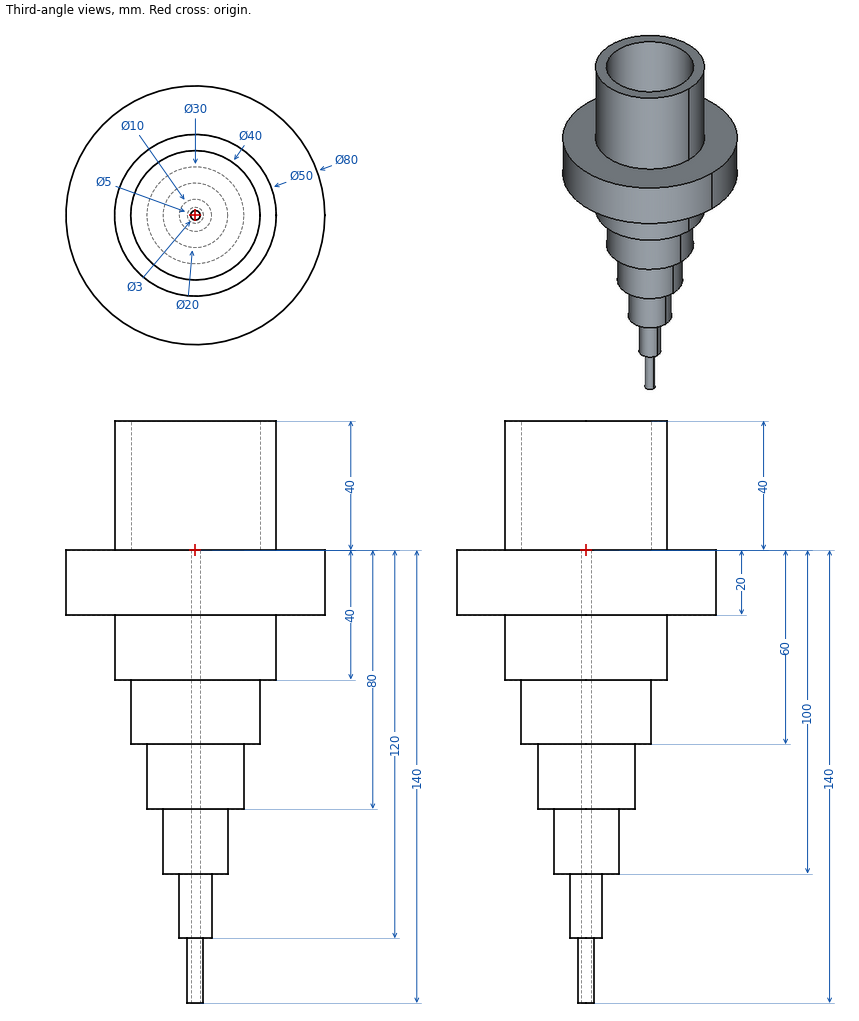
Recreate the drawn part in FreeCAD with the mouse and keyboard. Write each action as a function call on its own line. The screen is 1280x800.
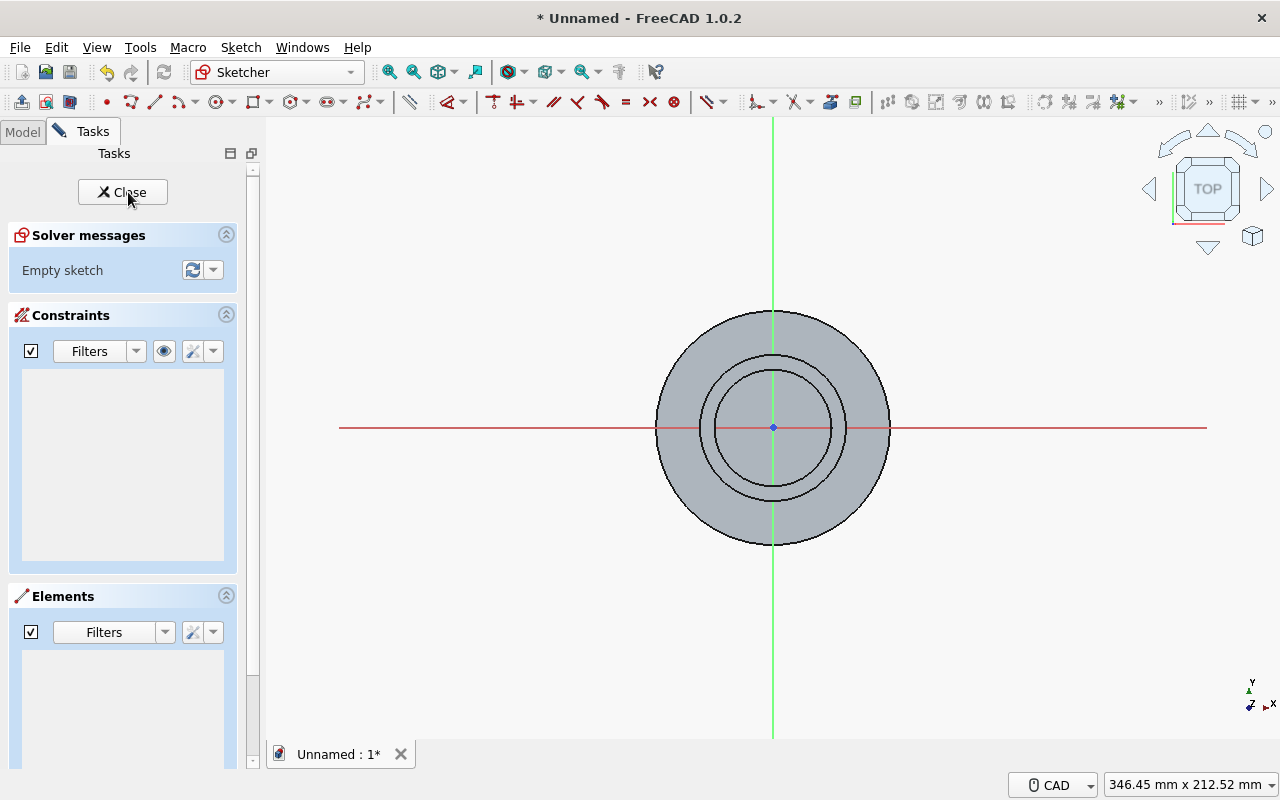
key(q)
key(s)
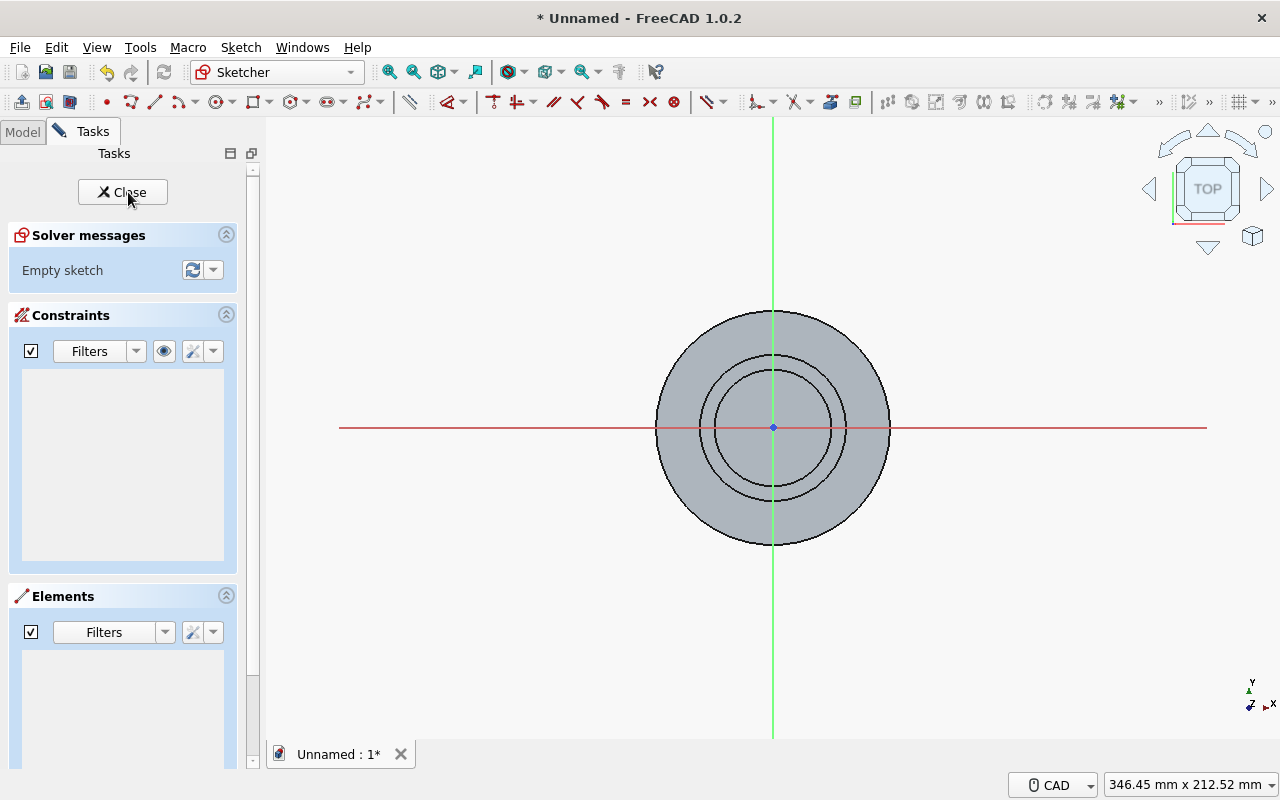
scroll(777, 428, up, 15)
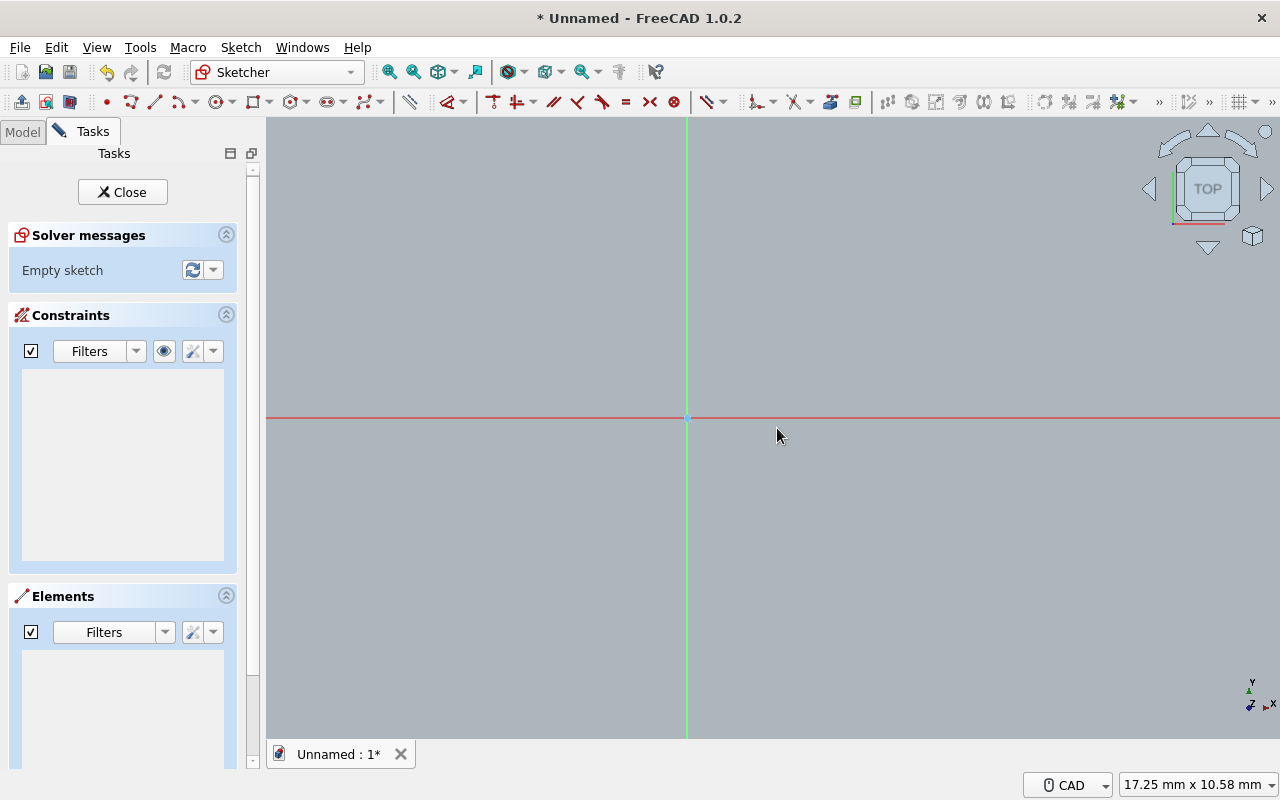
scroll(673, 411, up, 4)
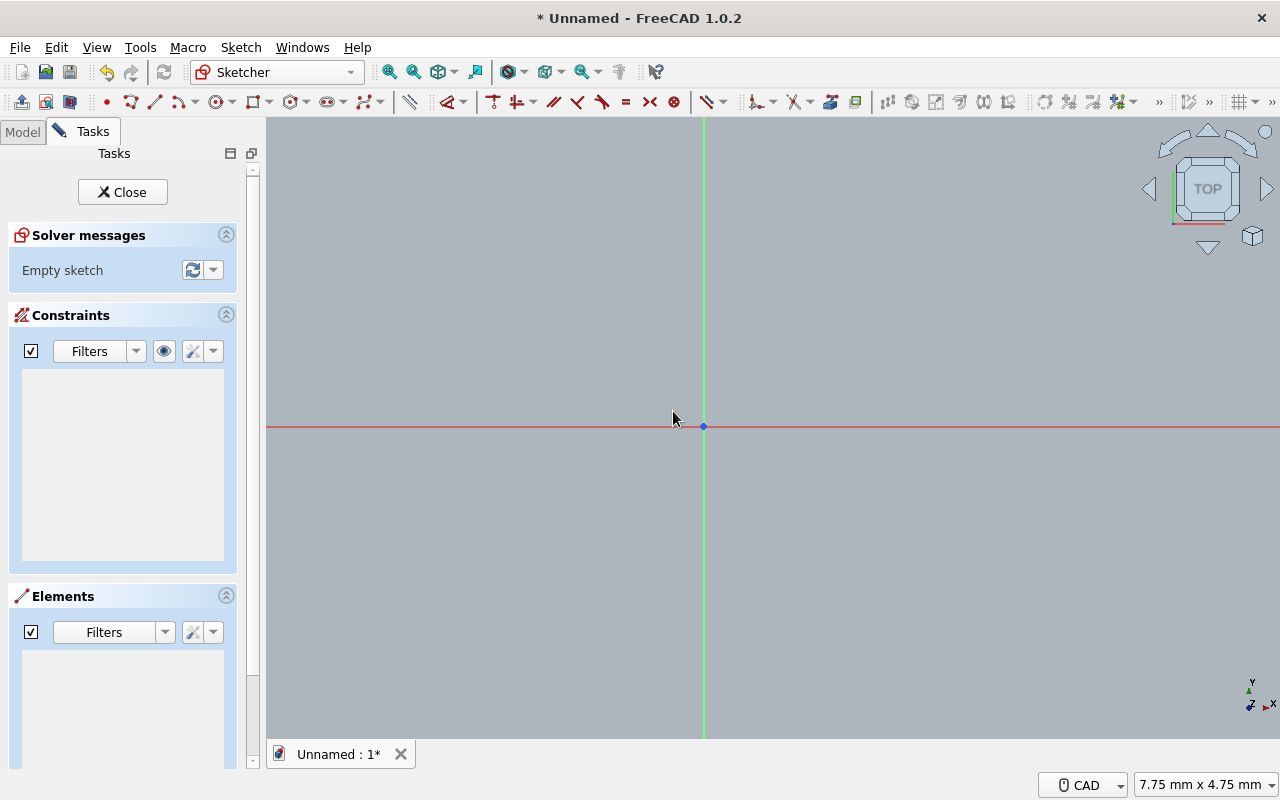
click(216, 102)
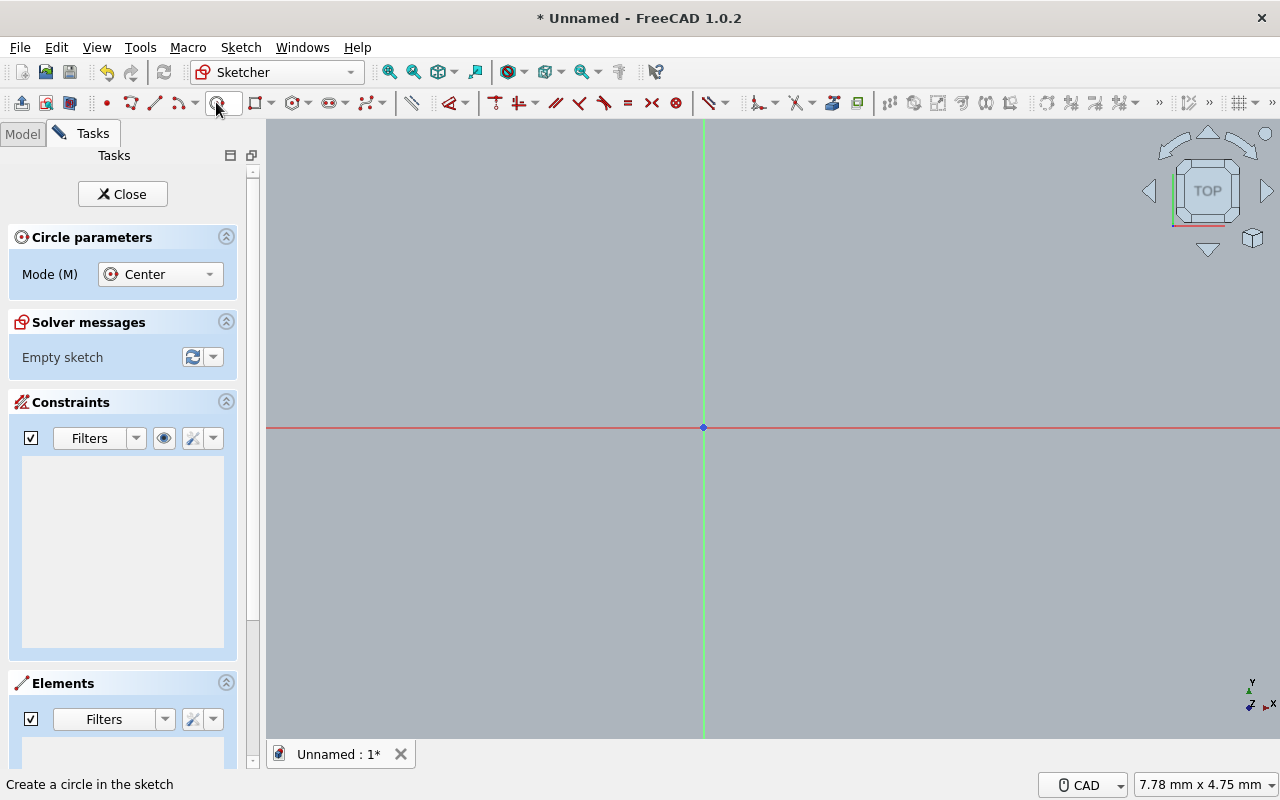
click(704, 428)
move(842, 290)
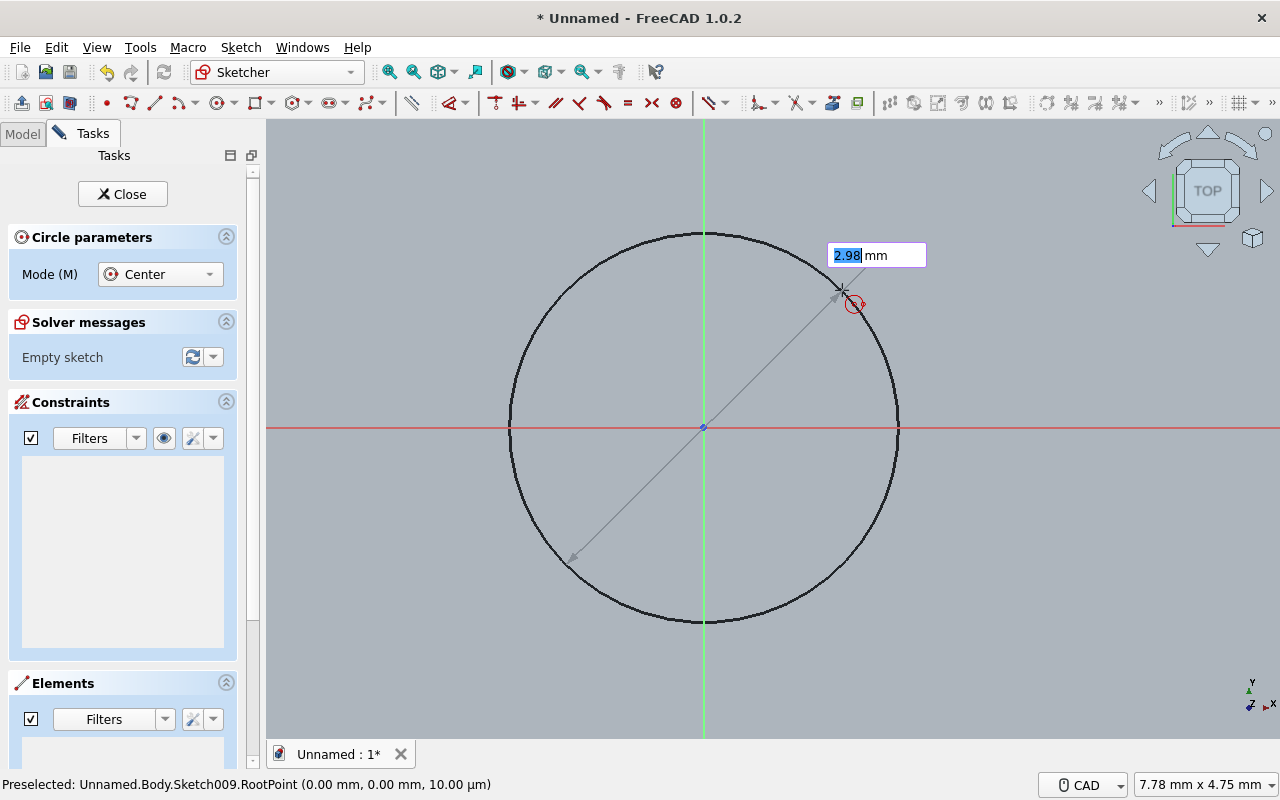
text(3)
key(Return)
key(Escape)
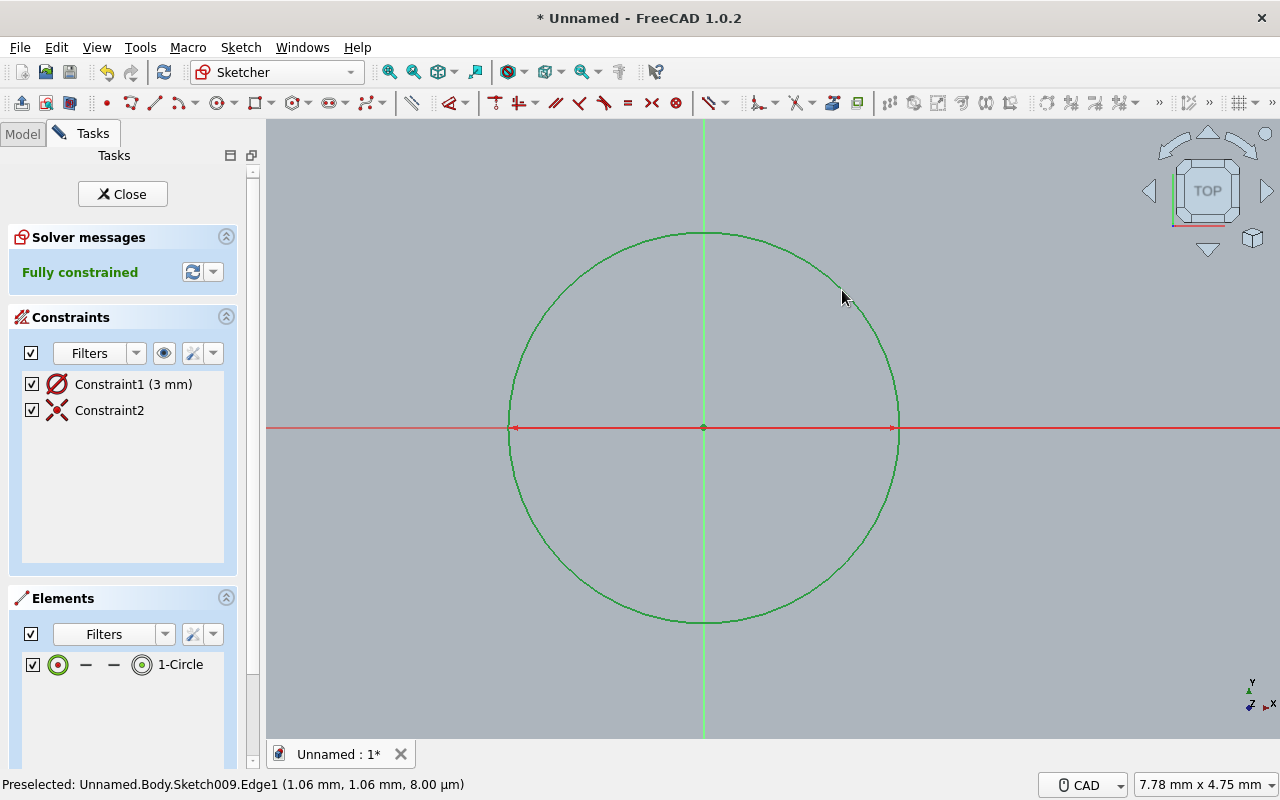
click(123, 194)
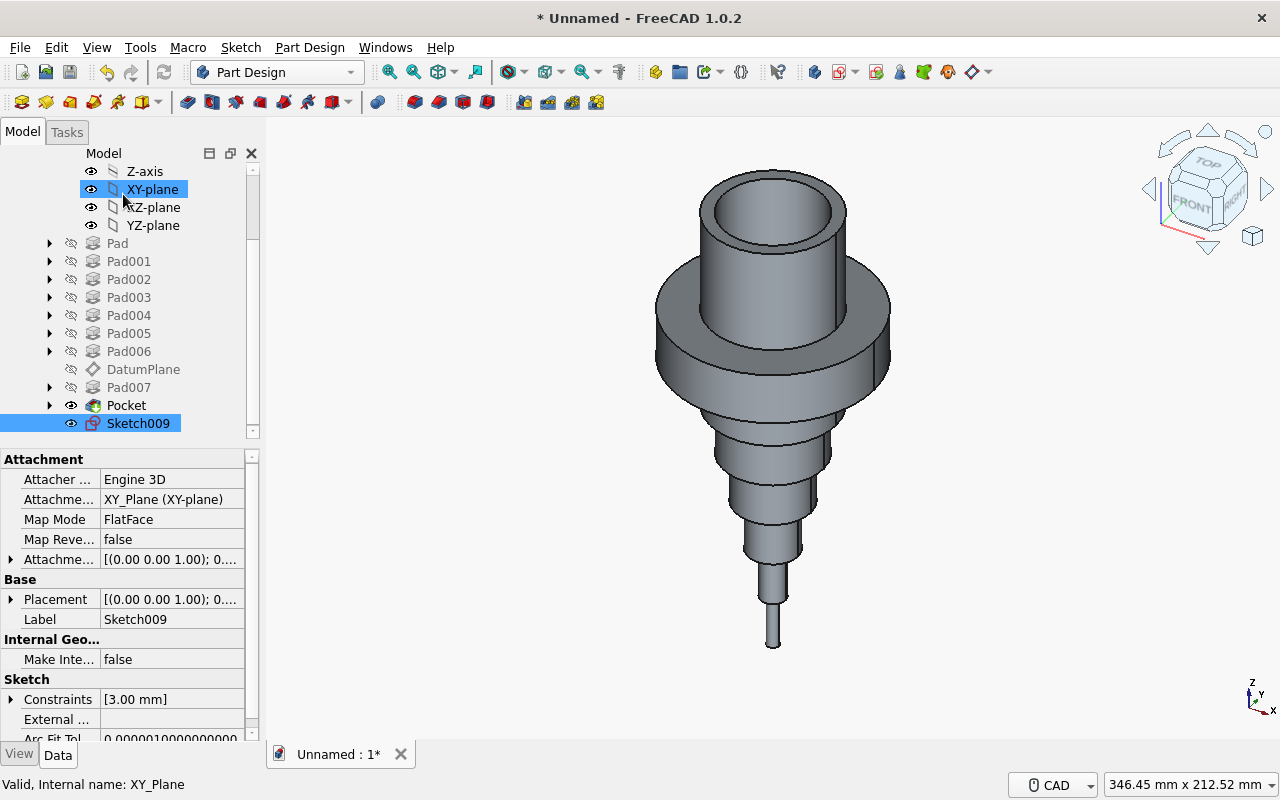
click(188, 102)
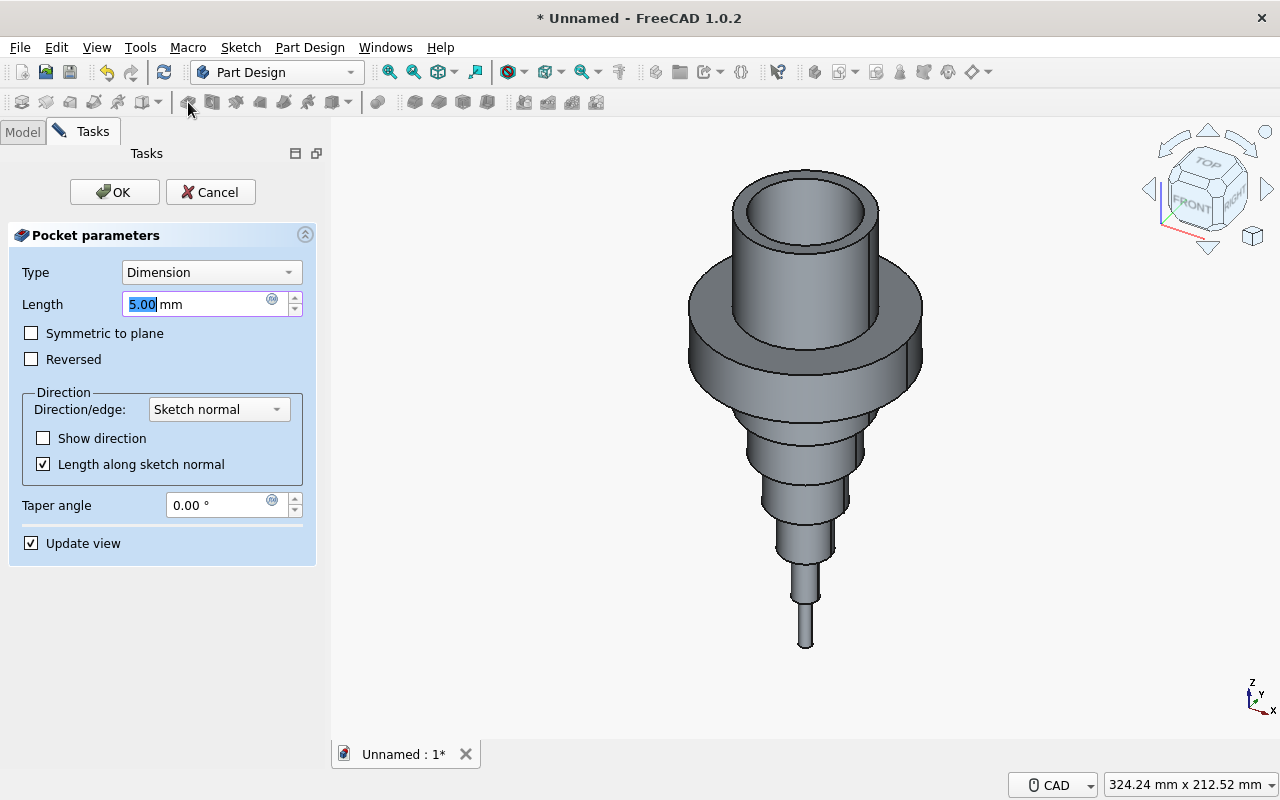
text(140)
key(Tab)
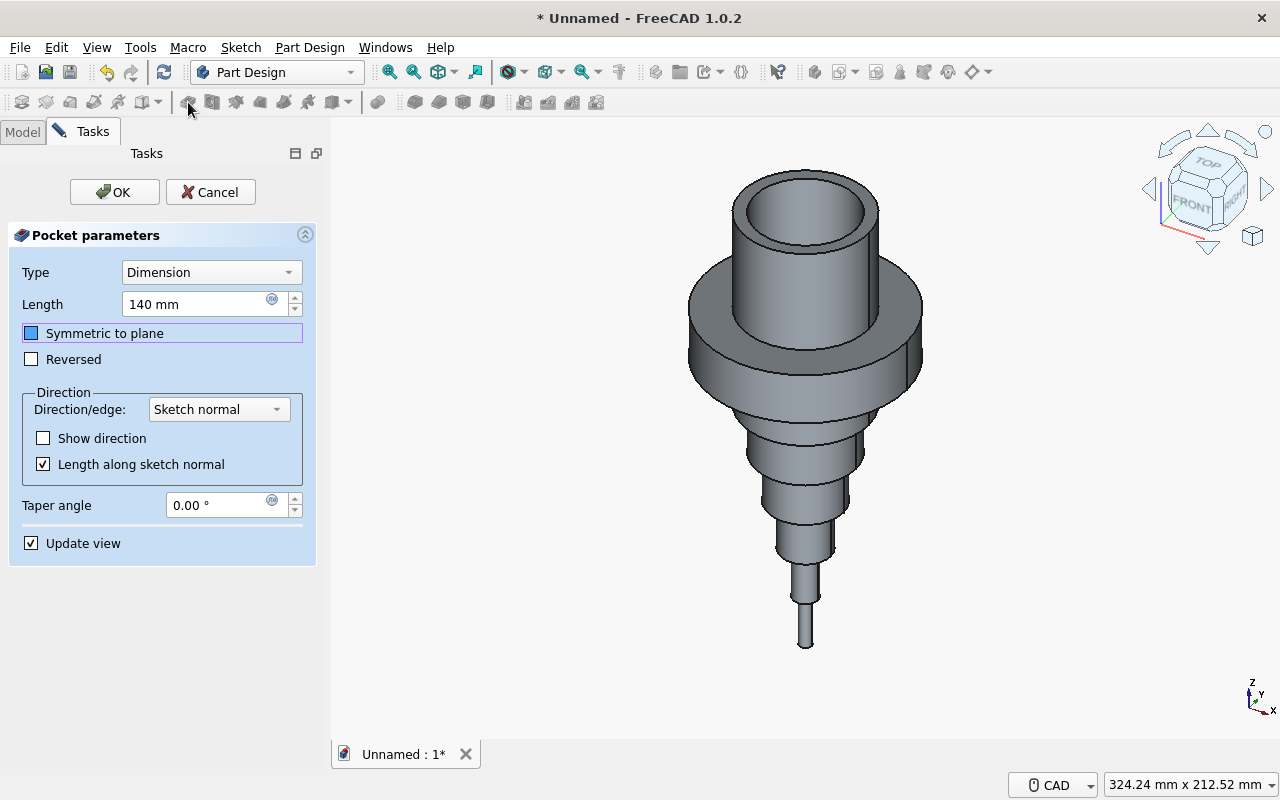
click(115, 192)